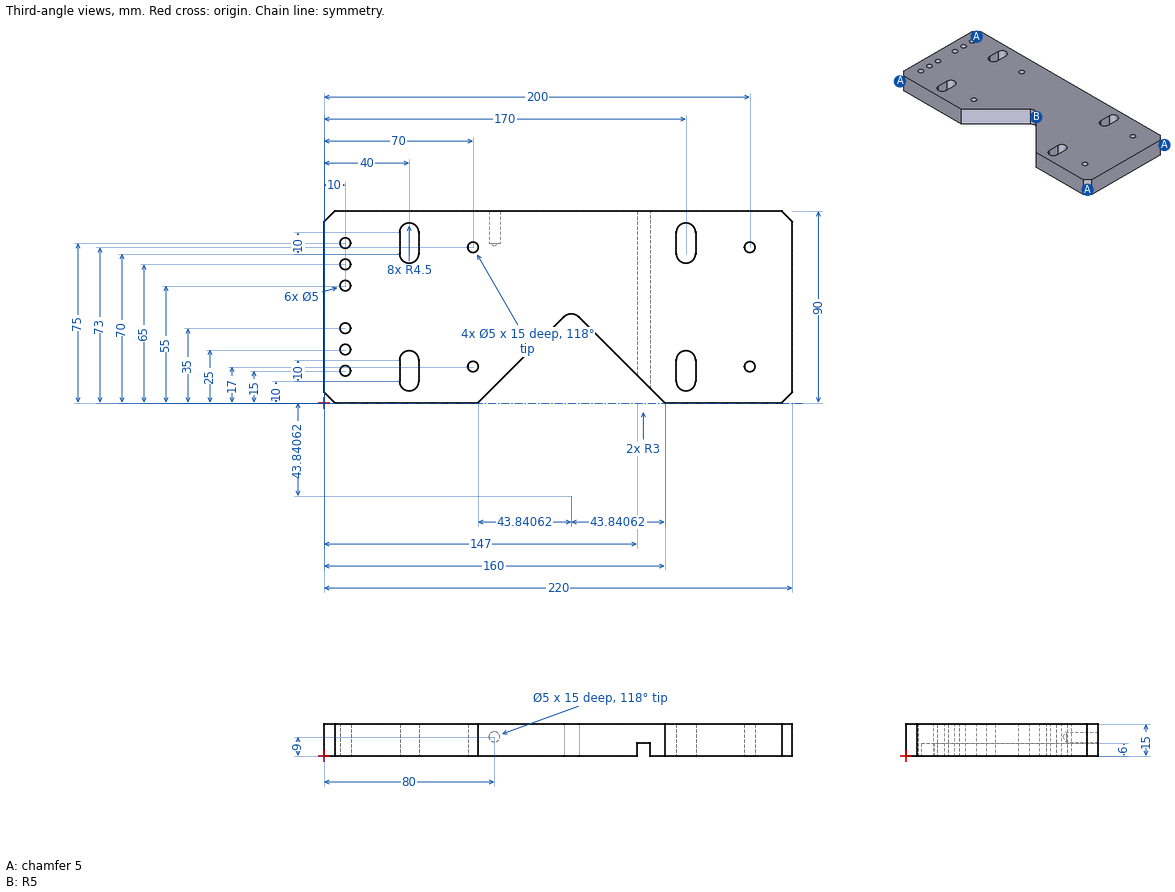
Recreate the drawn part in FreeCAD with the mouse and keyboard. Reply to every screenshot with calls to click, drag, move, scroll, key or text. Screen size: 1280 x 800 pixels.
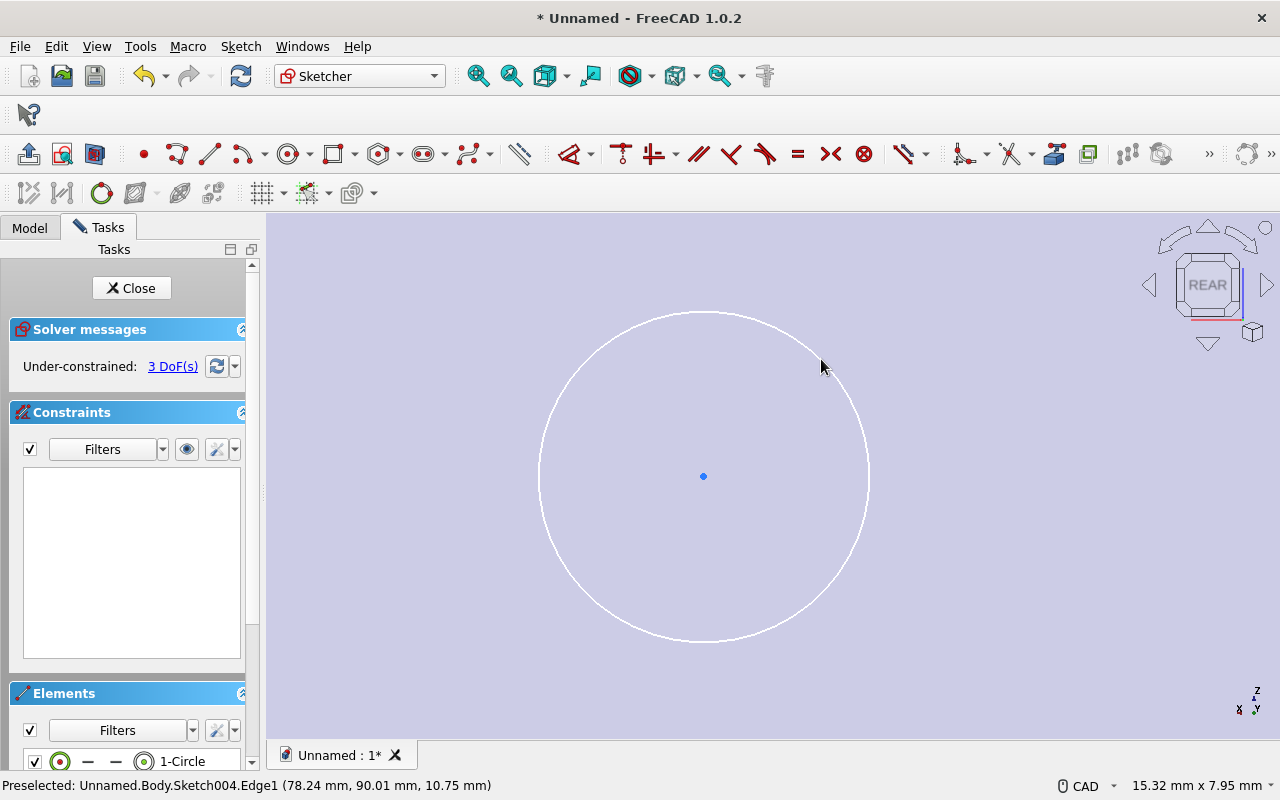
key(d)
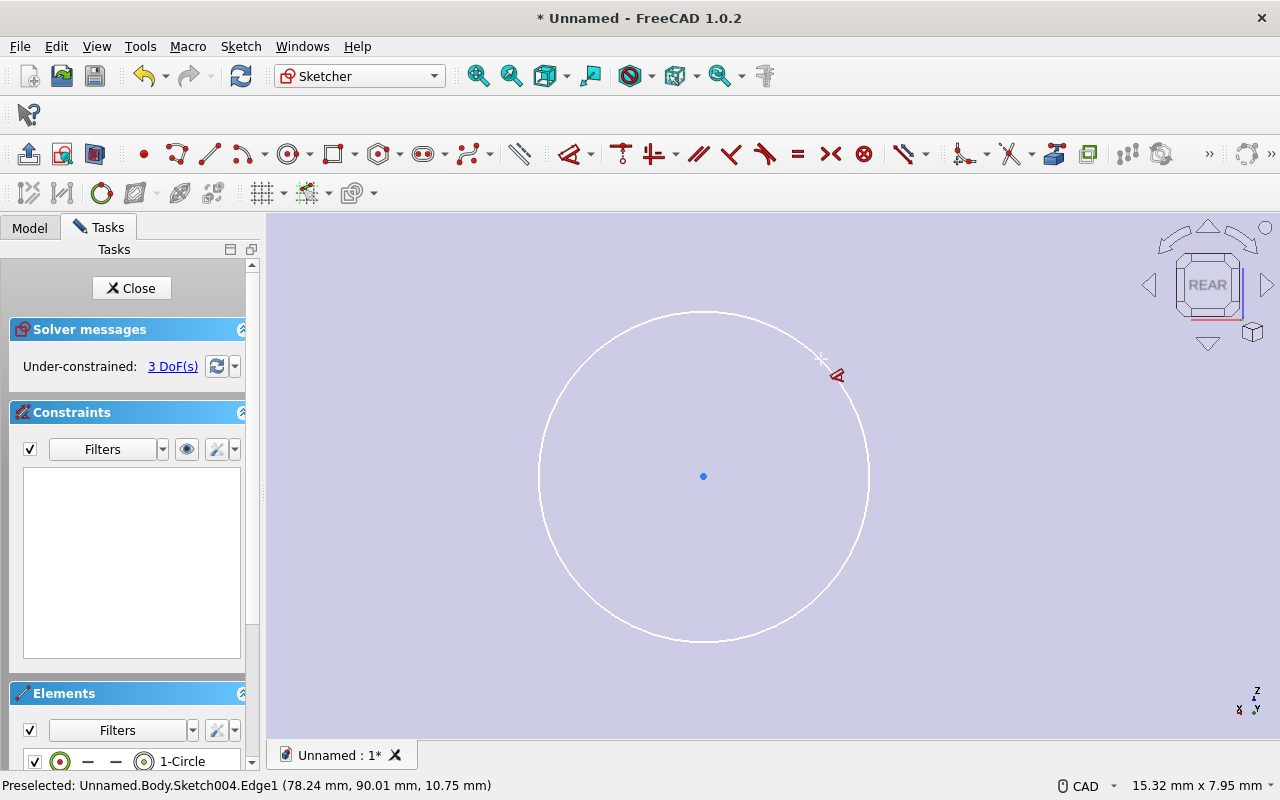
click(821, 360)
click(844, 337)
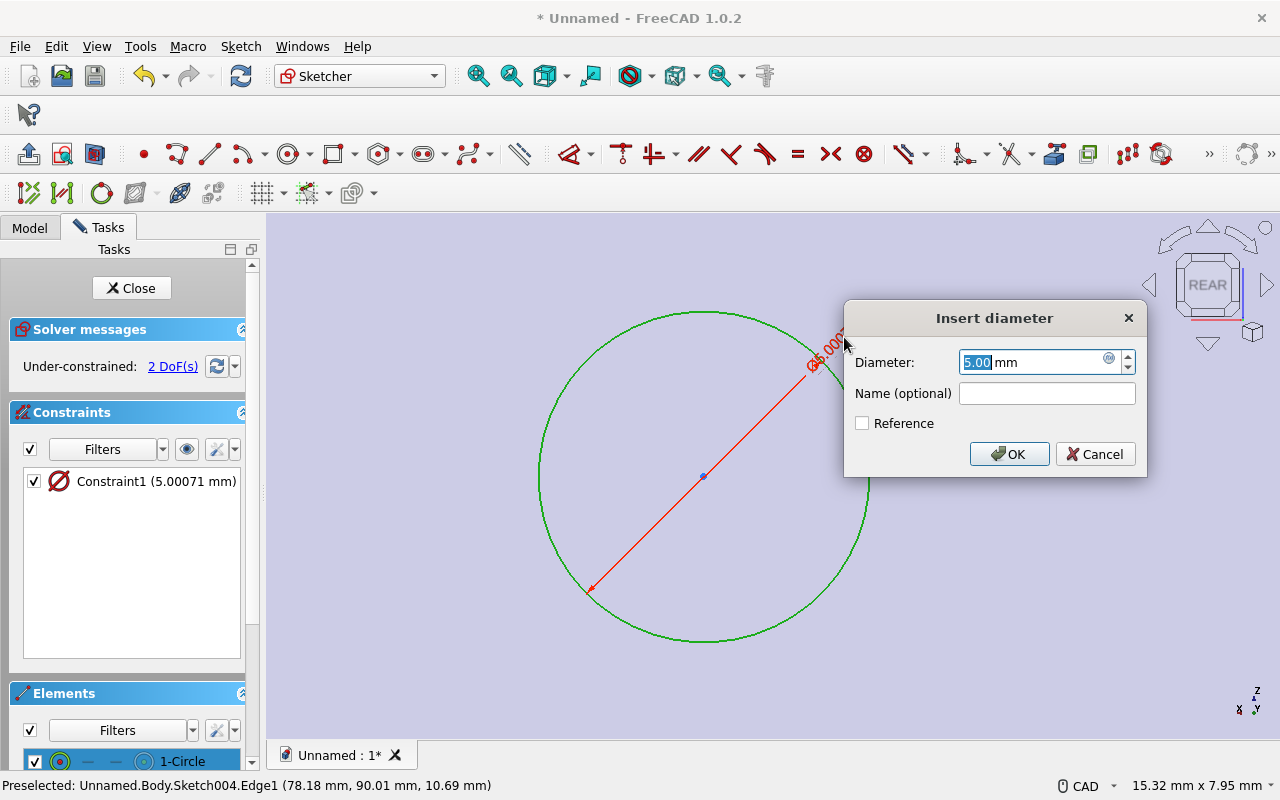
text(5)
key(Return)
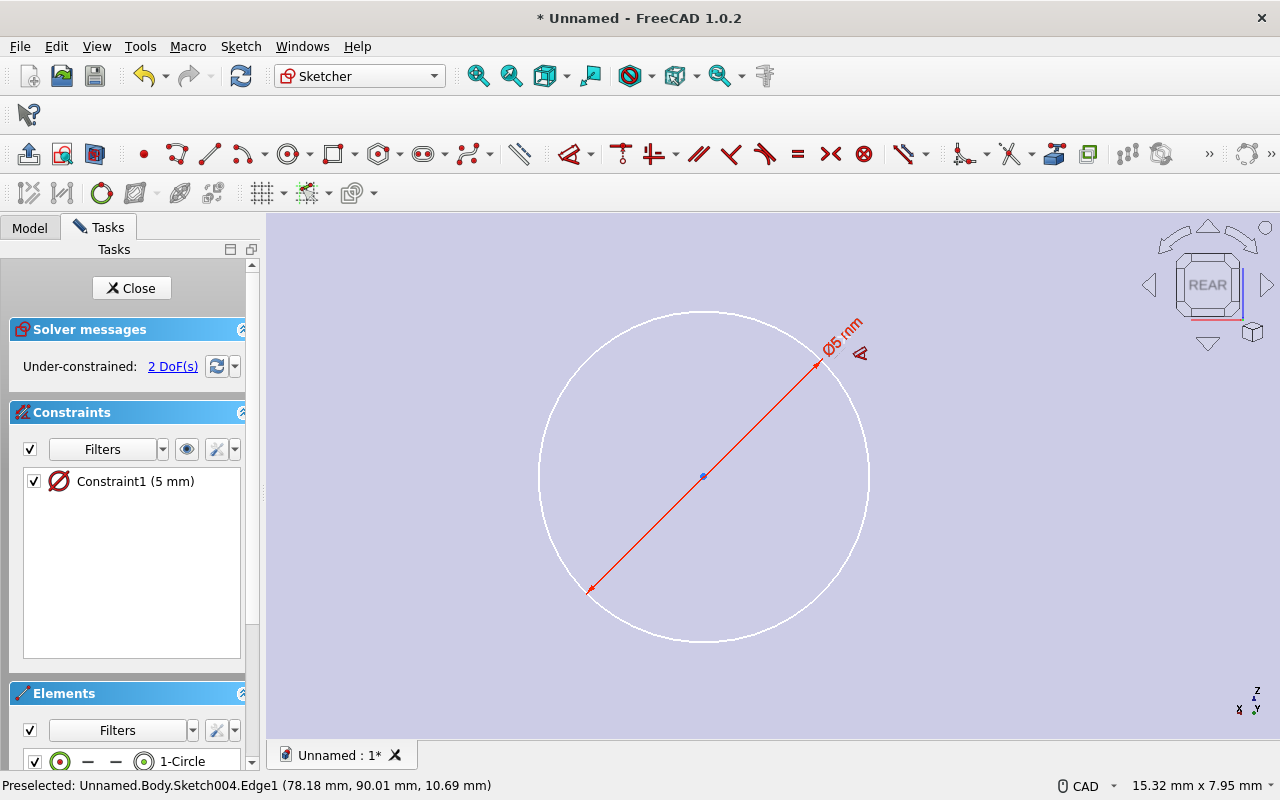
click(704, 477)
click(670, 594)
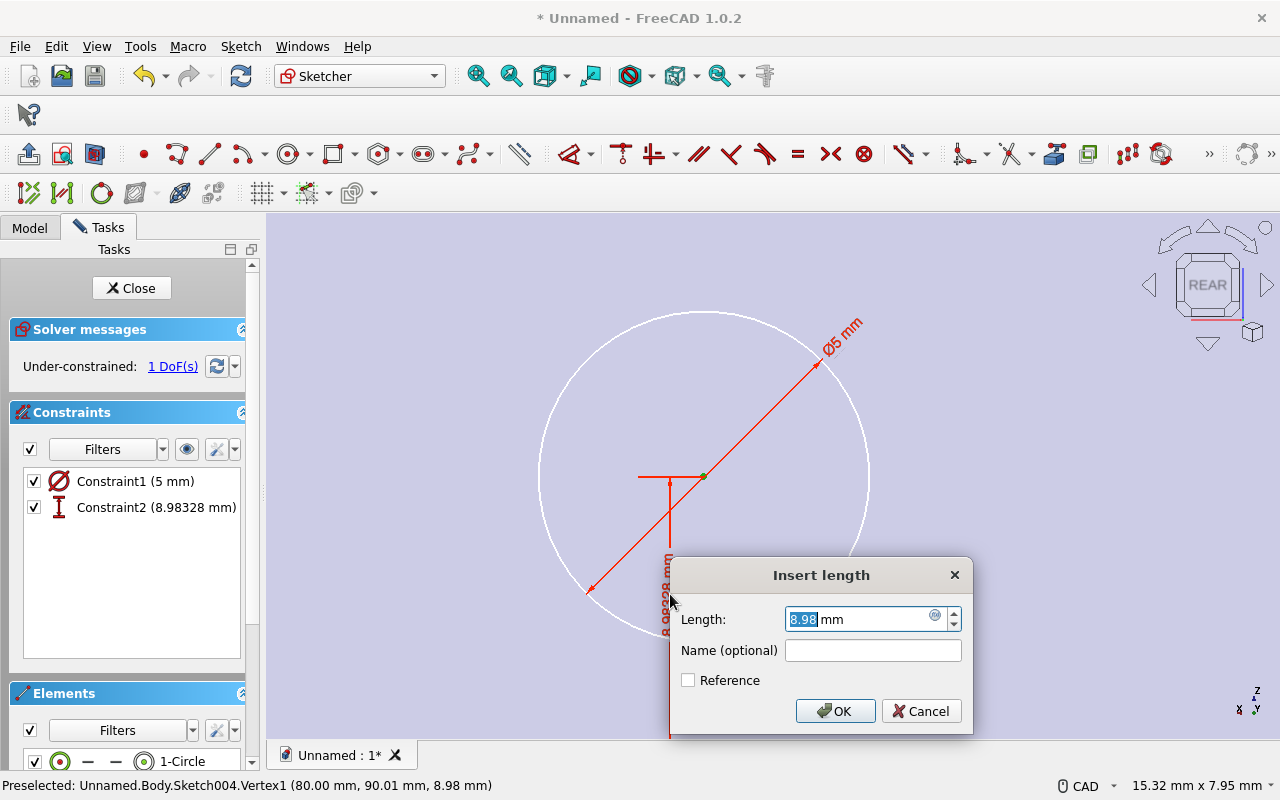
text(9)
key(Return)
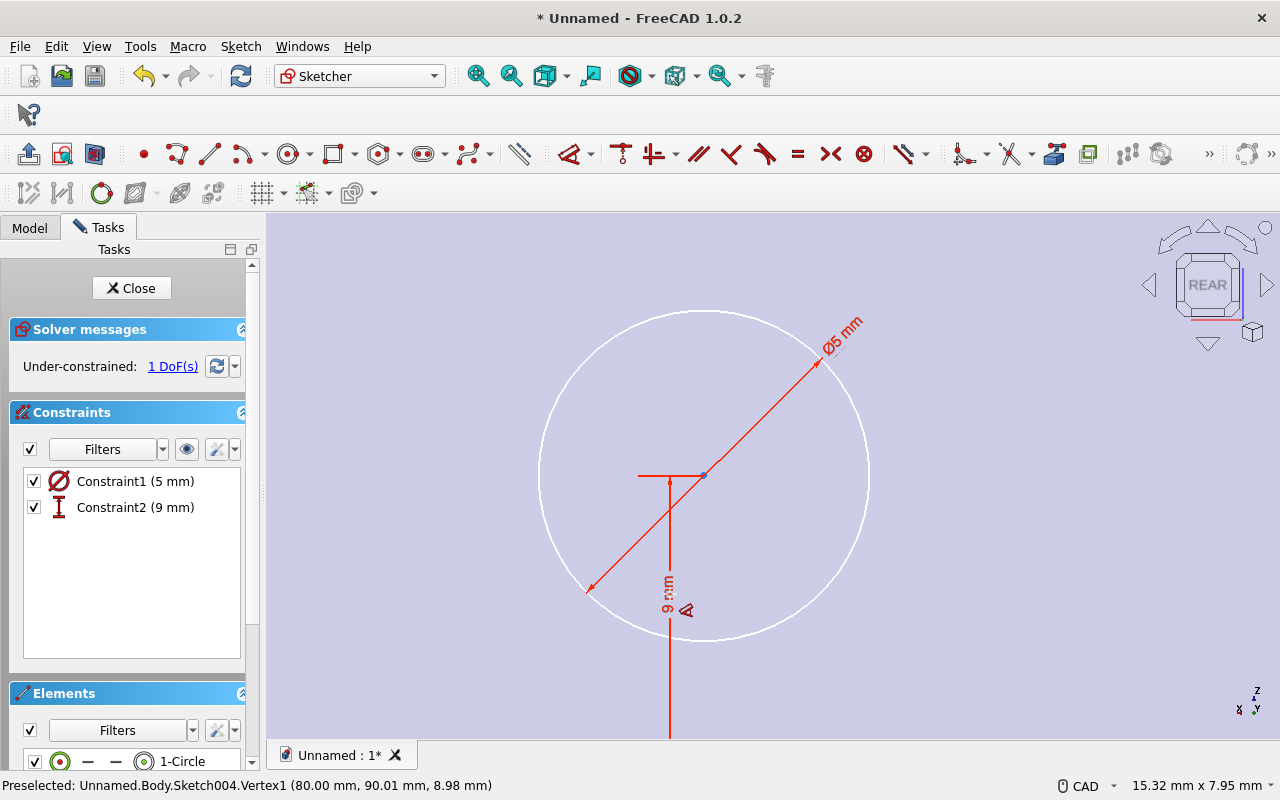
click(704, 476)
click(909, 442)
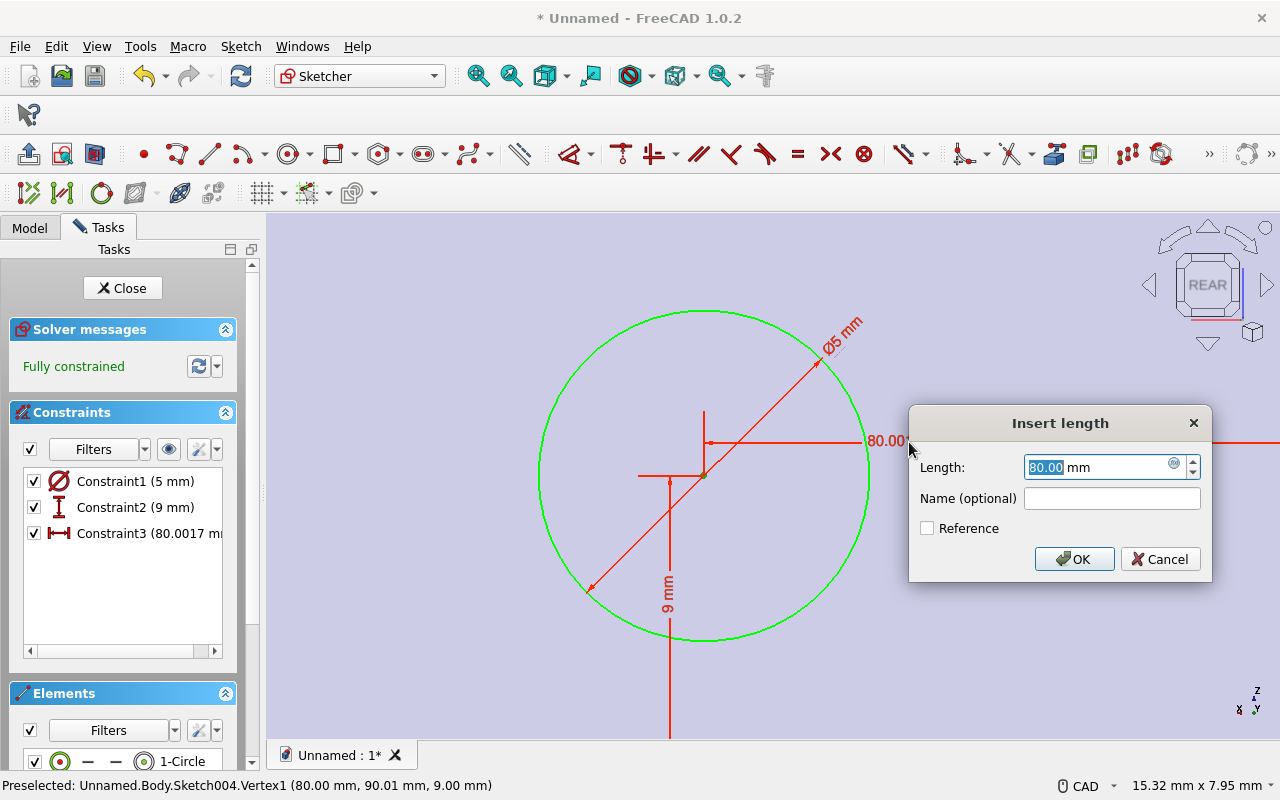
text(80)
key(Return)
key(Escape)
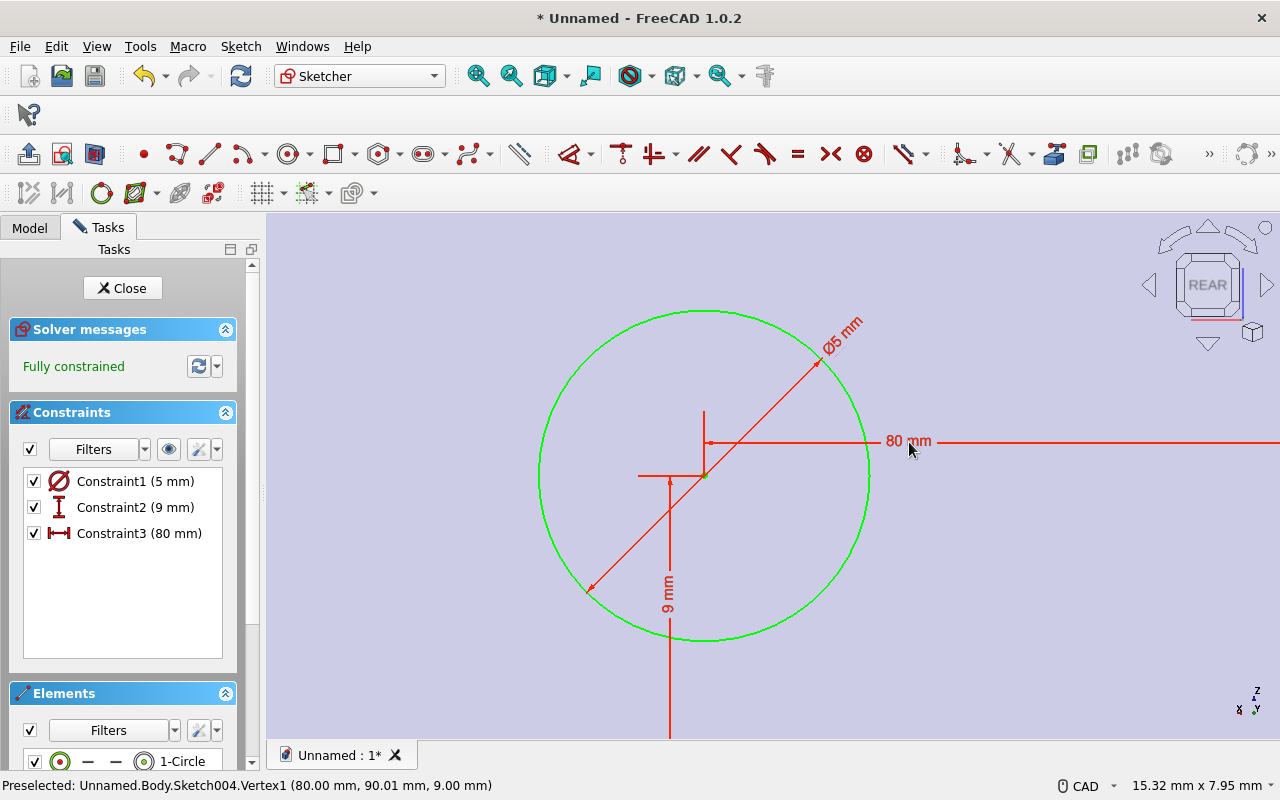
click(123, 288)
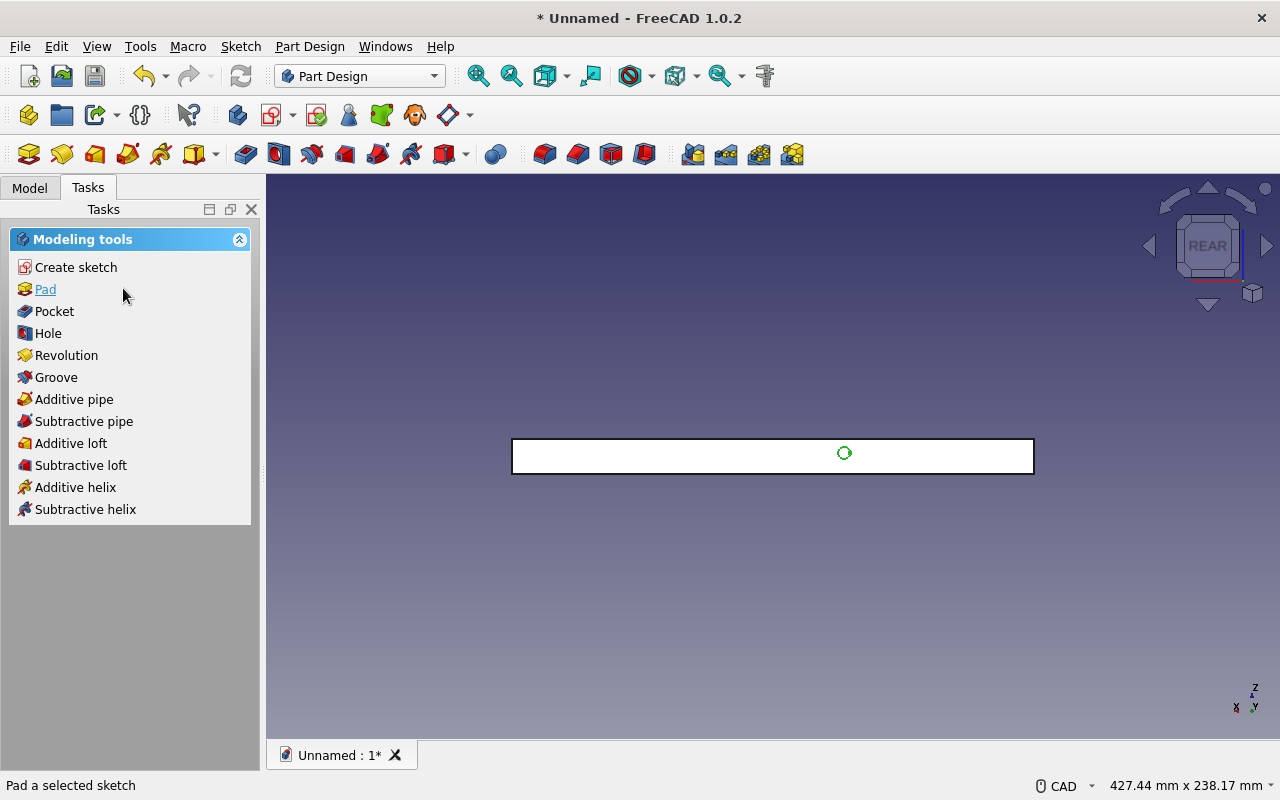
click(279, 154)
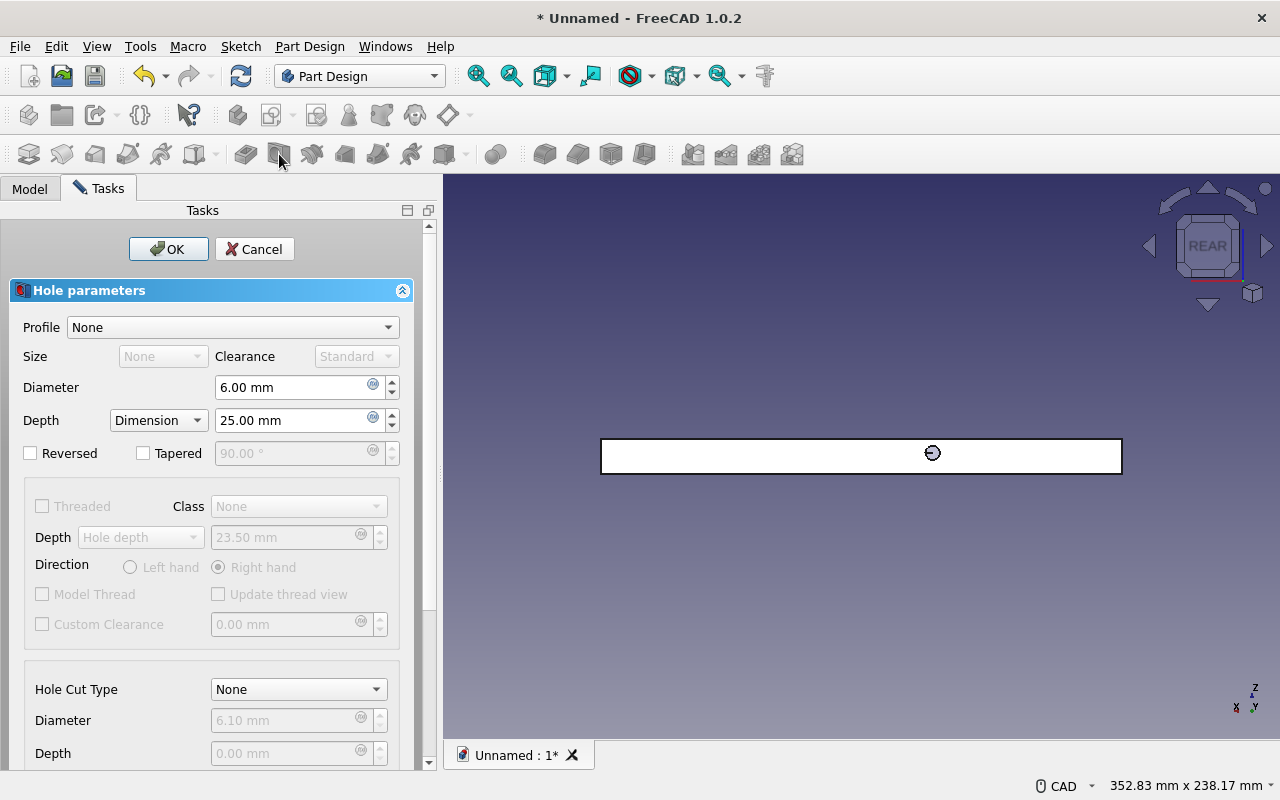
triple_click(300, 388)